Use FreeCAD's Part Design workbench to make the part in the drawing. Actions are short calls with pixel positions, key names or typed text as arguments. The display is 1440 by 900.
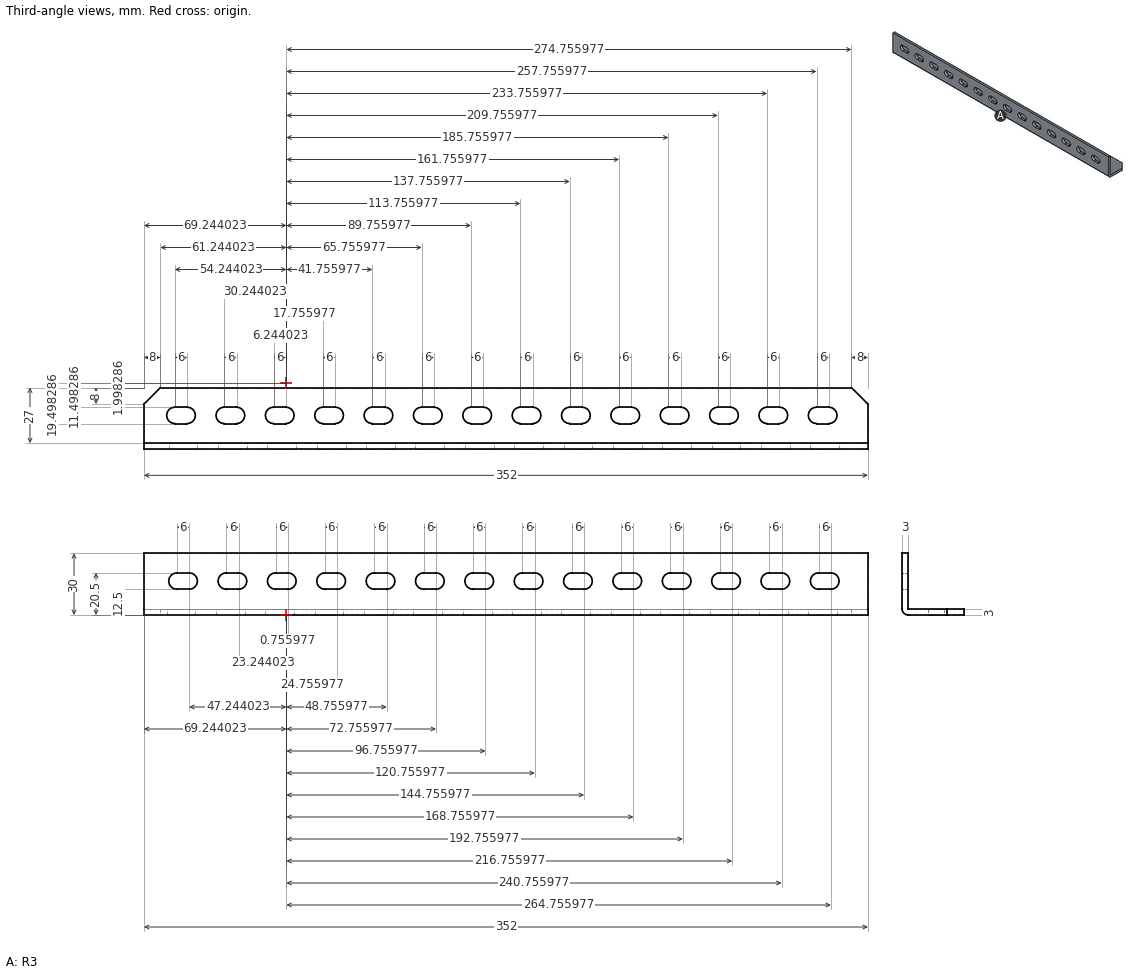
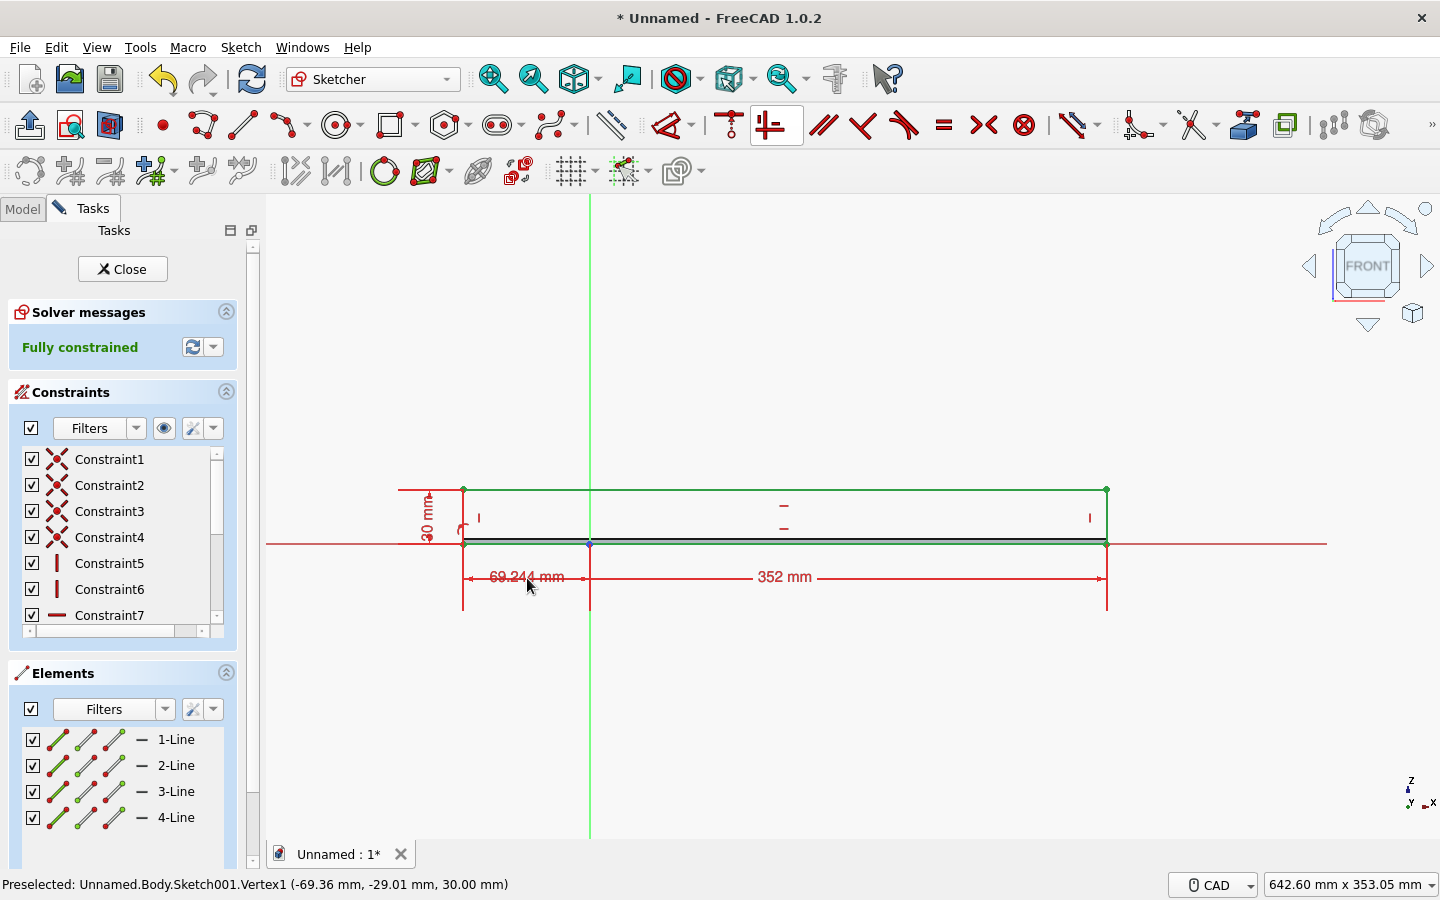
click(123, 269)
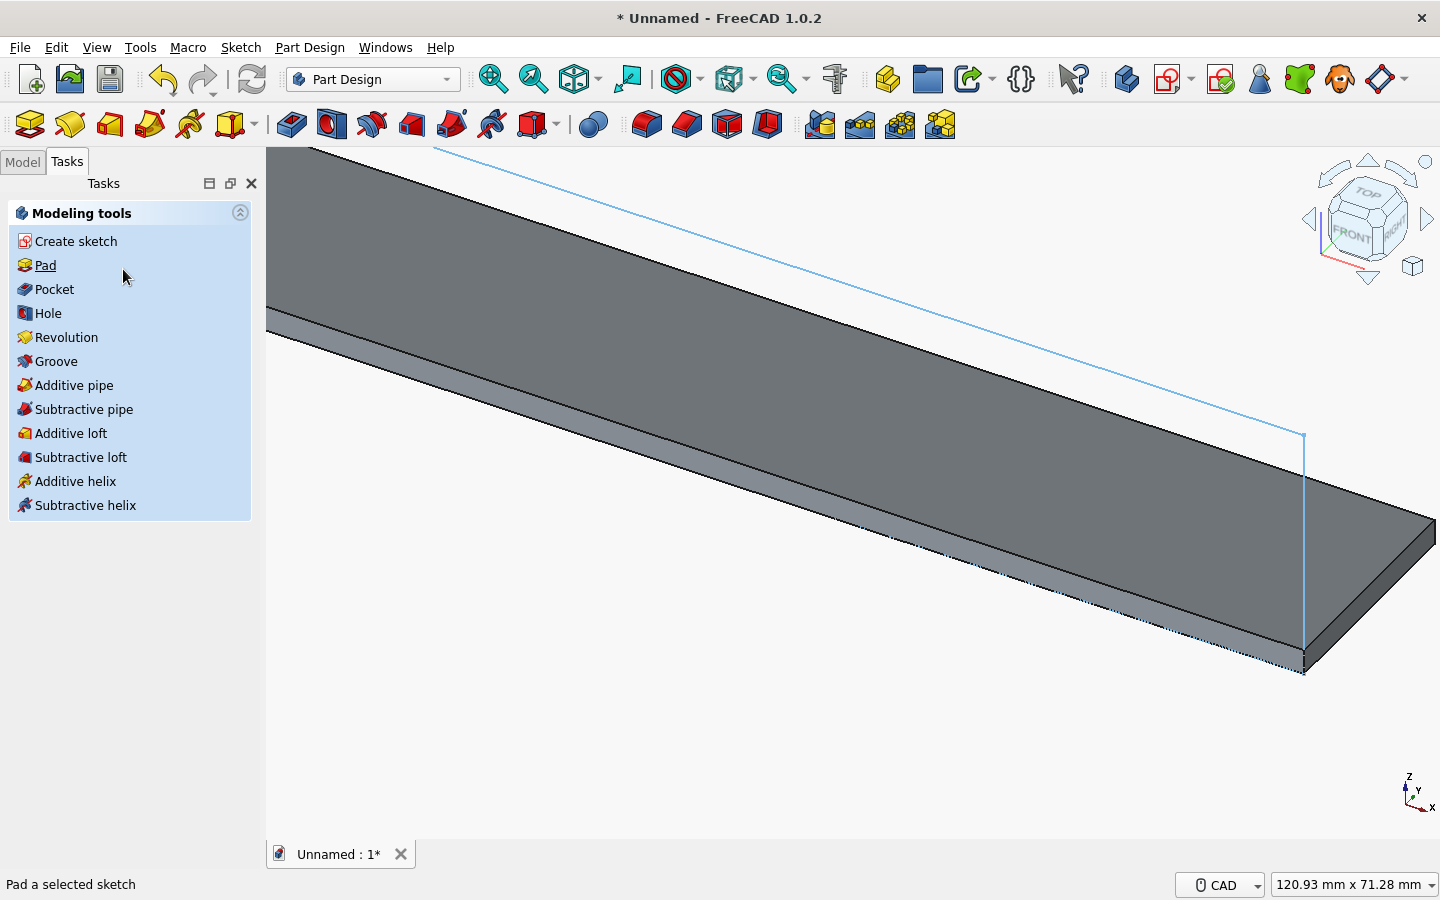
click(30, 124)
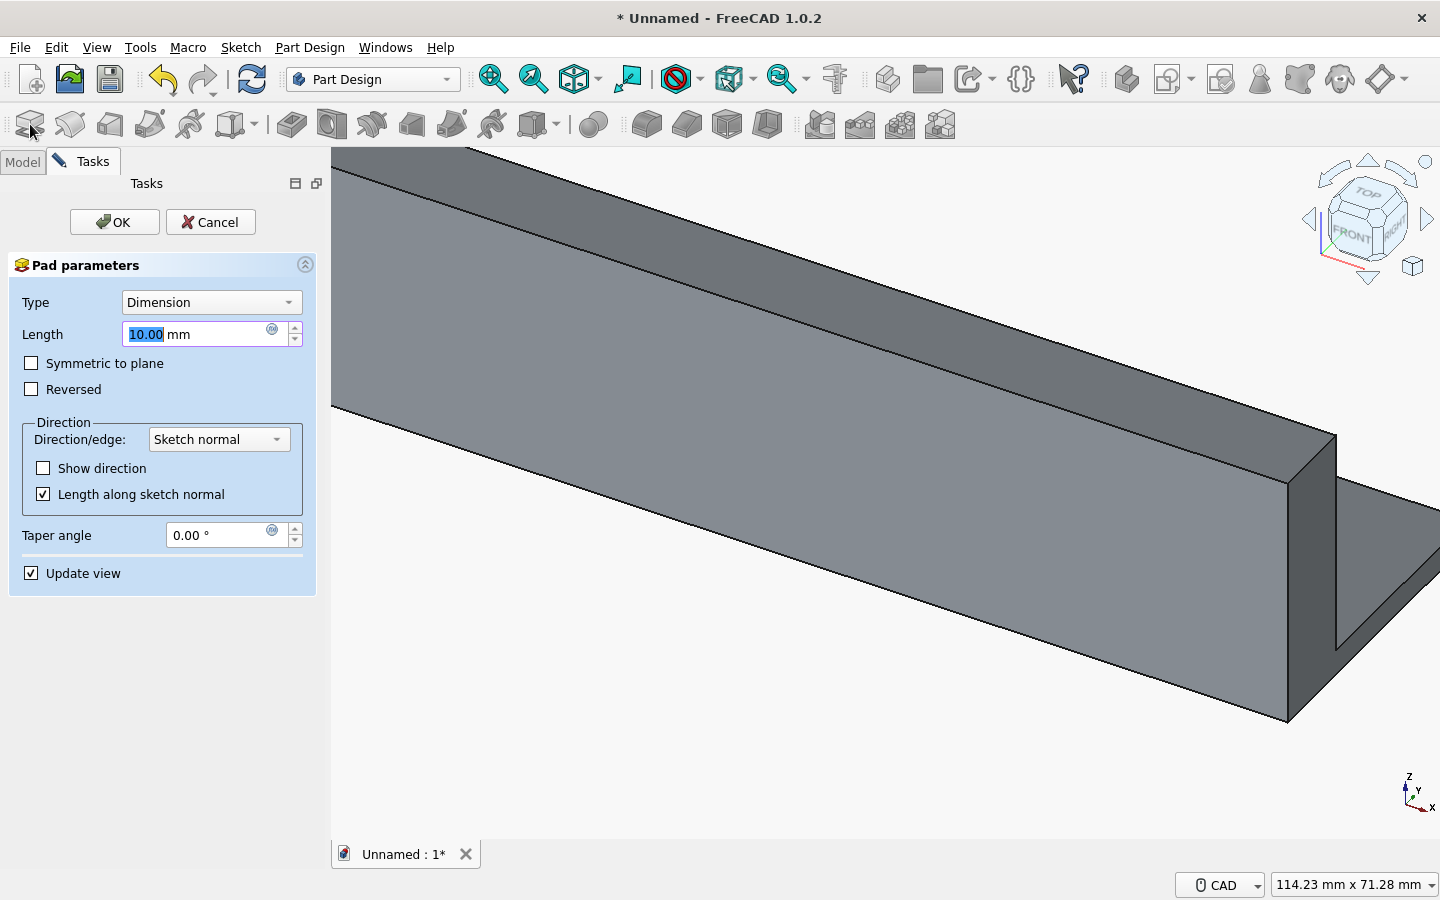
text(3)
key(Tab)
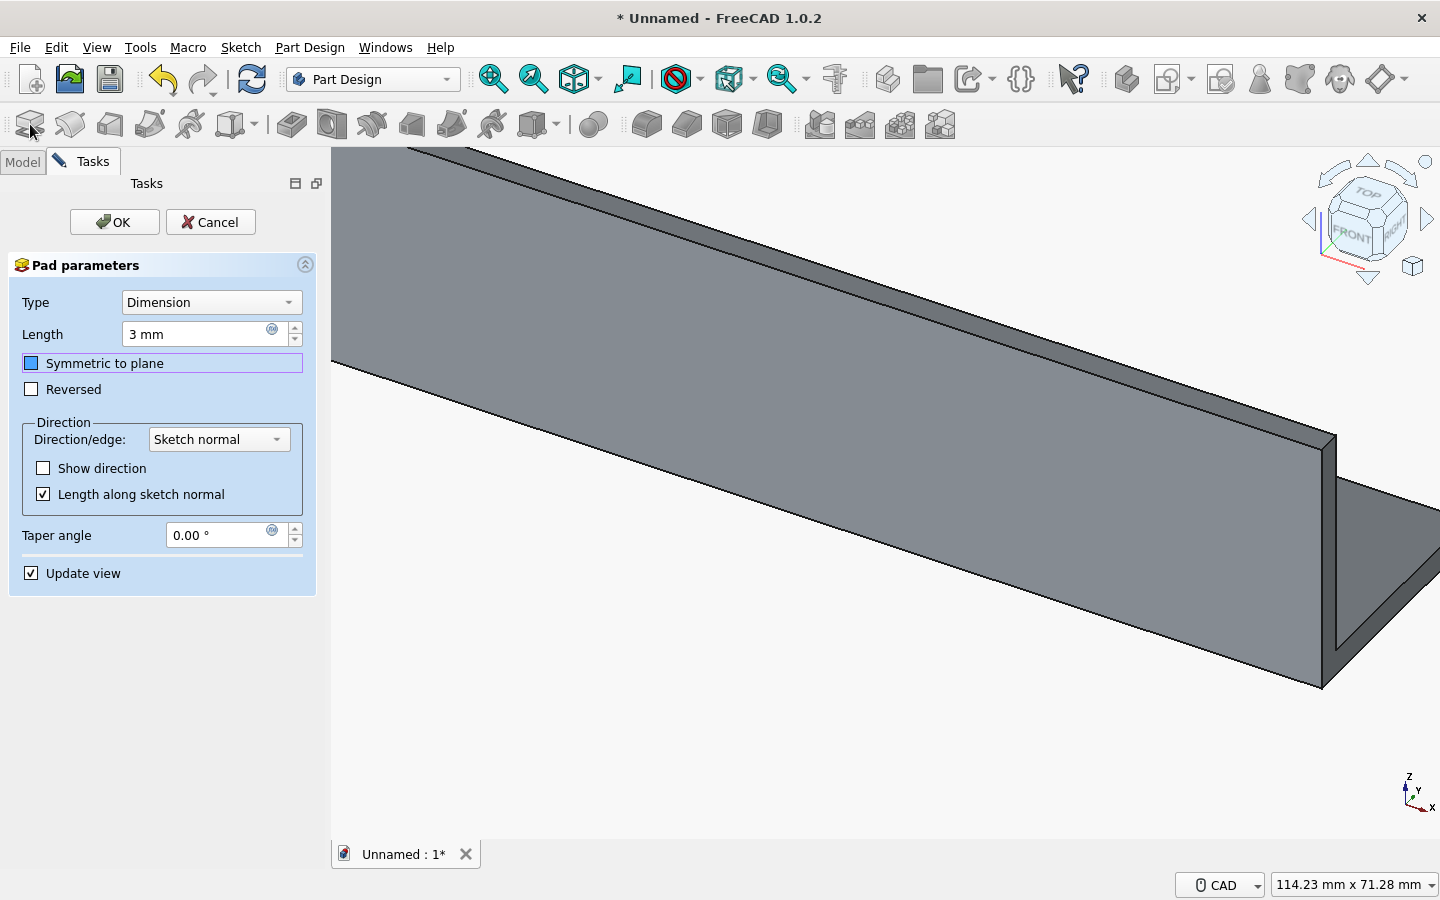
click(115, 222)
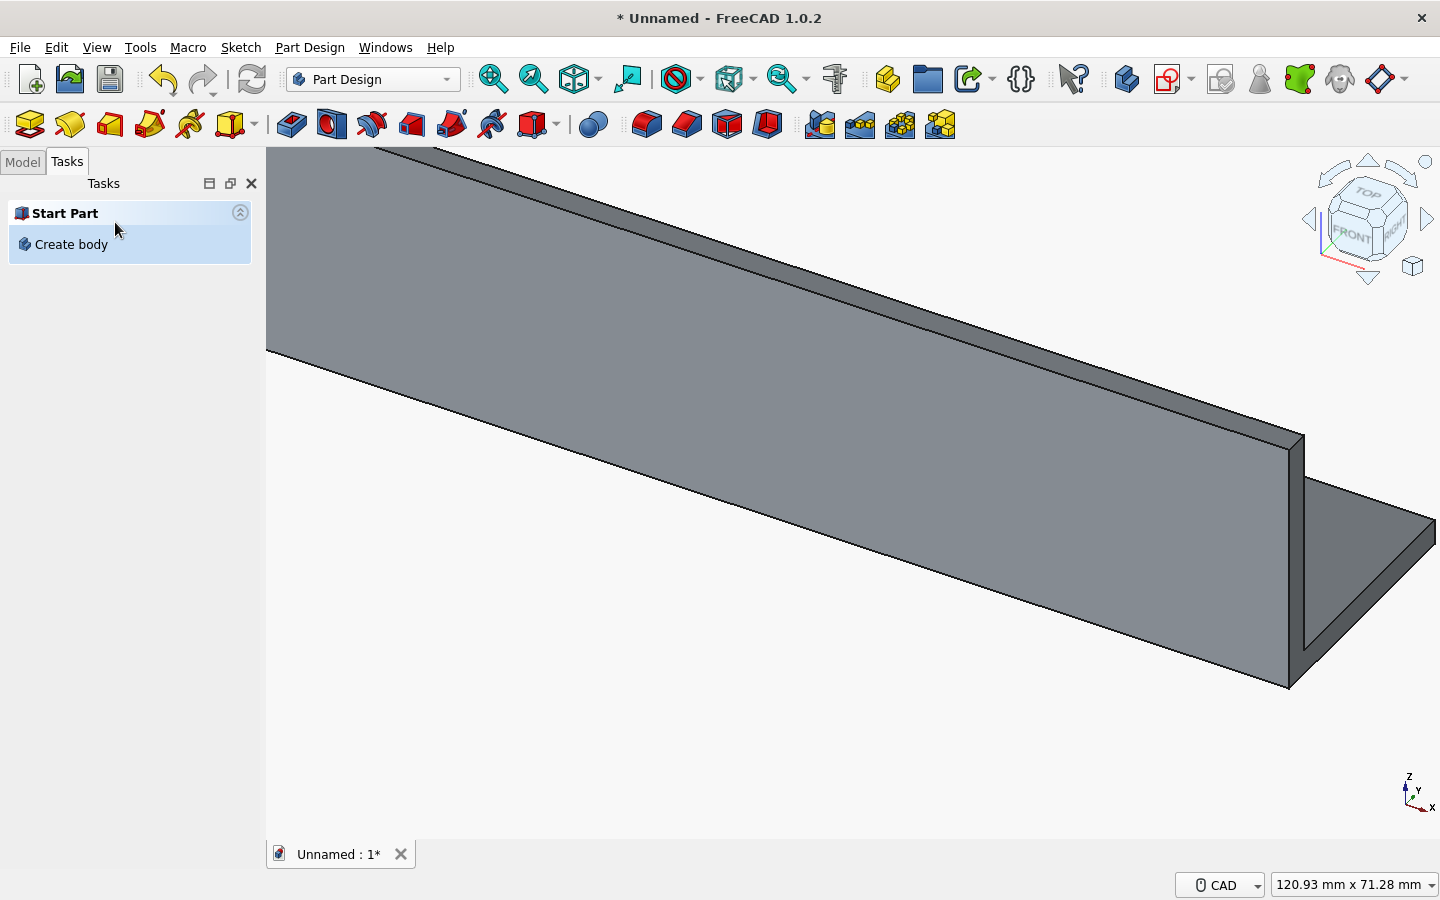
click(494, 80)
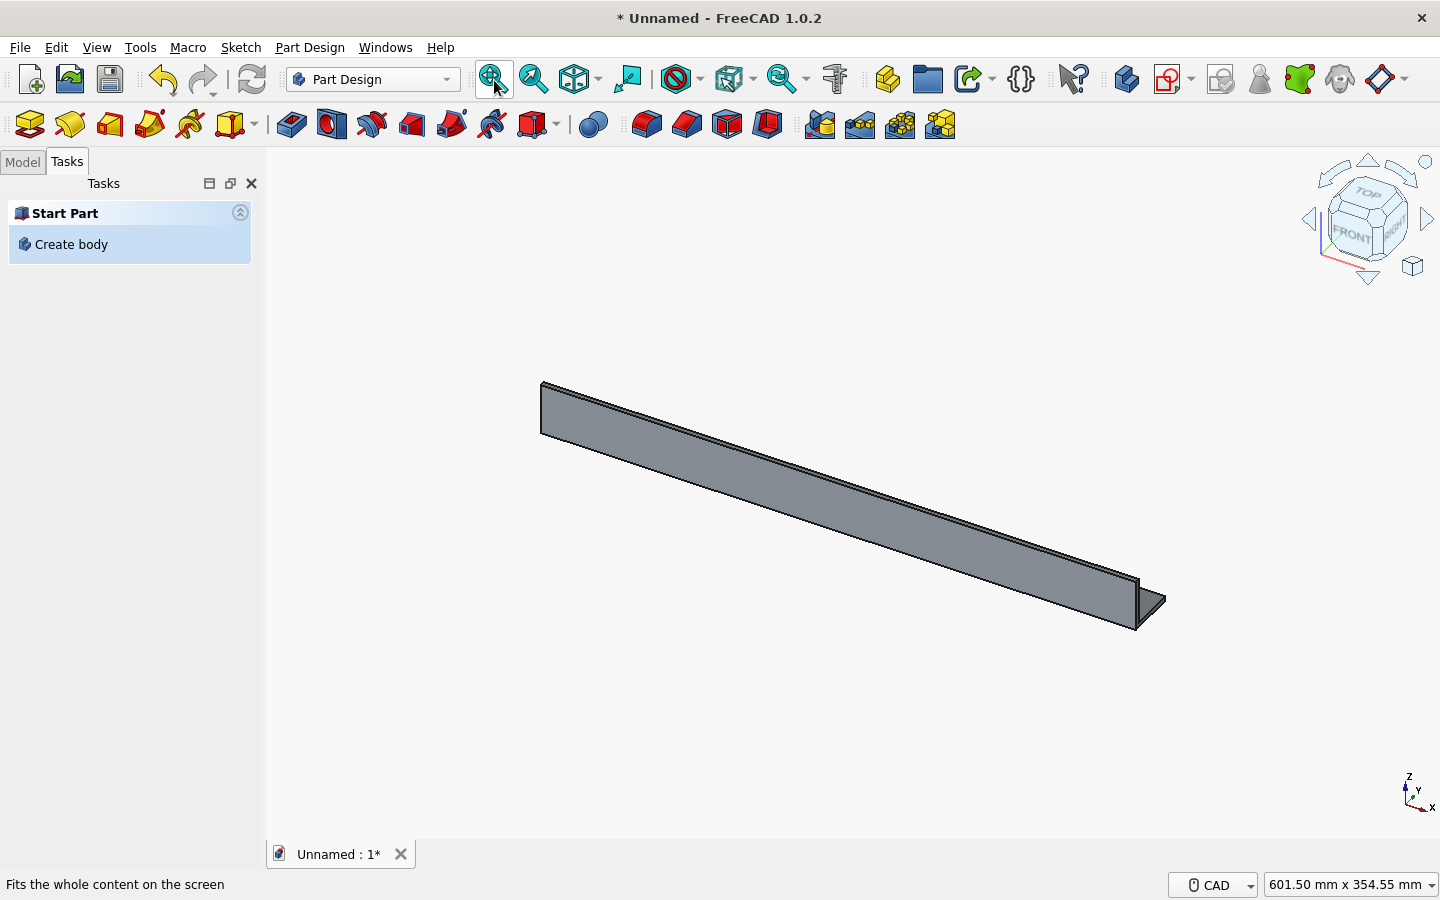
key(0)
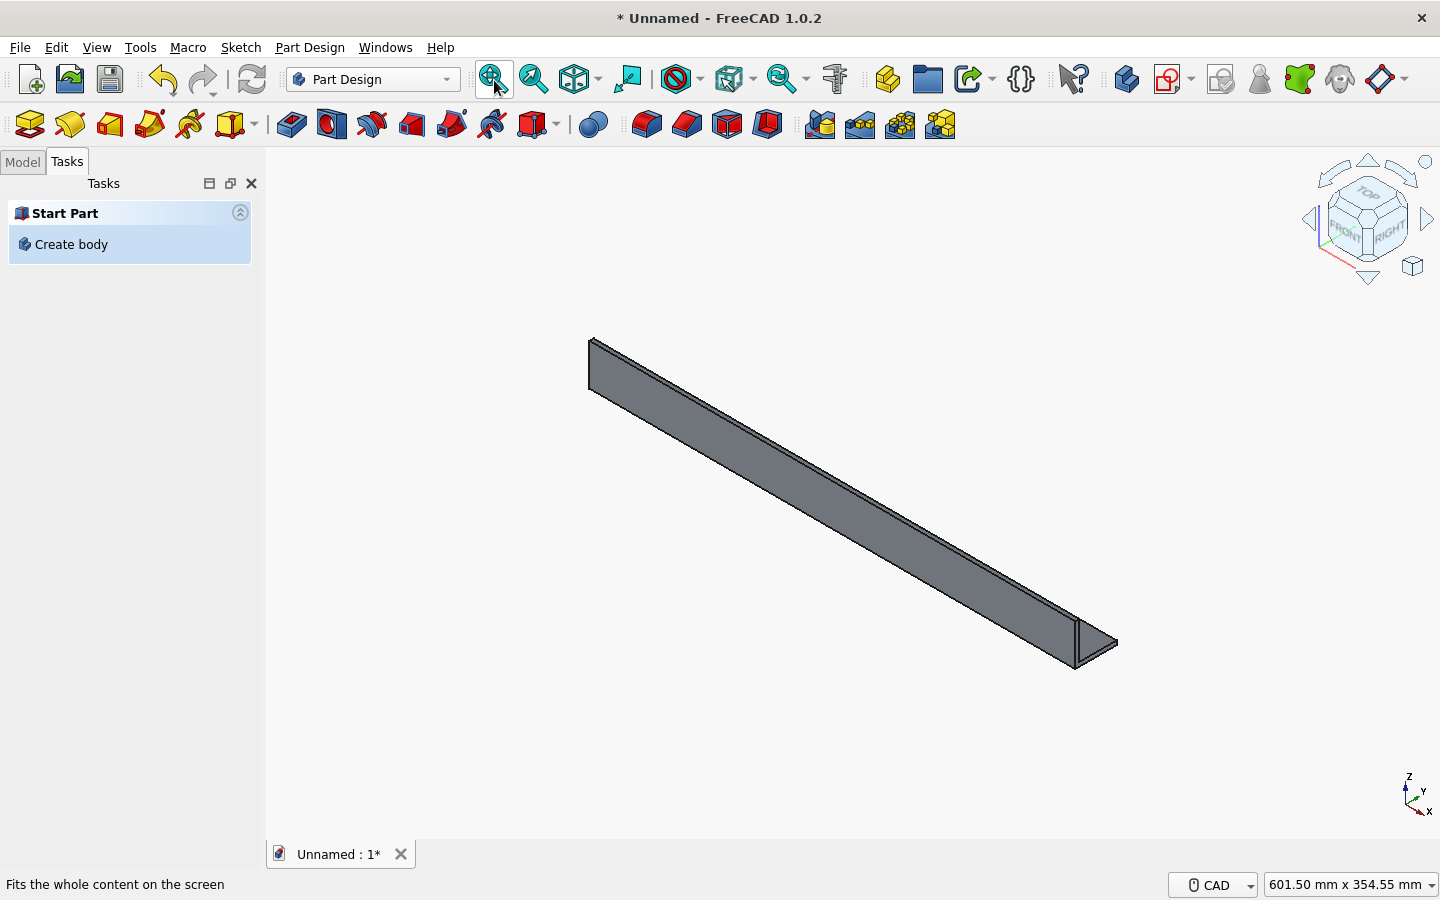
key(2)